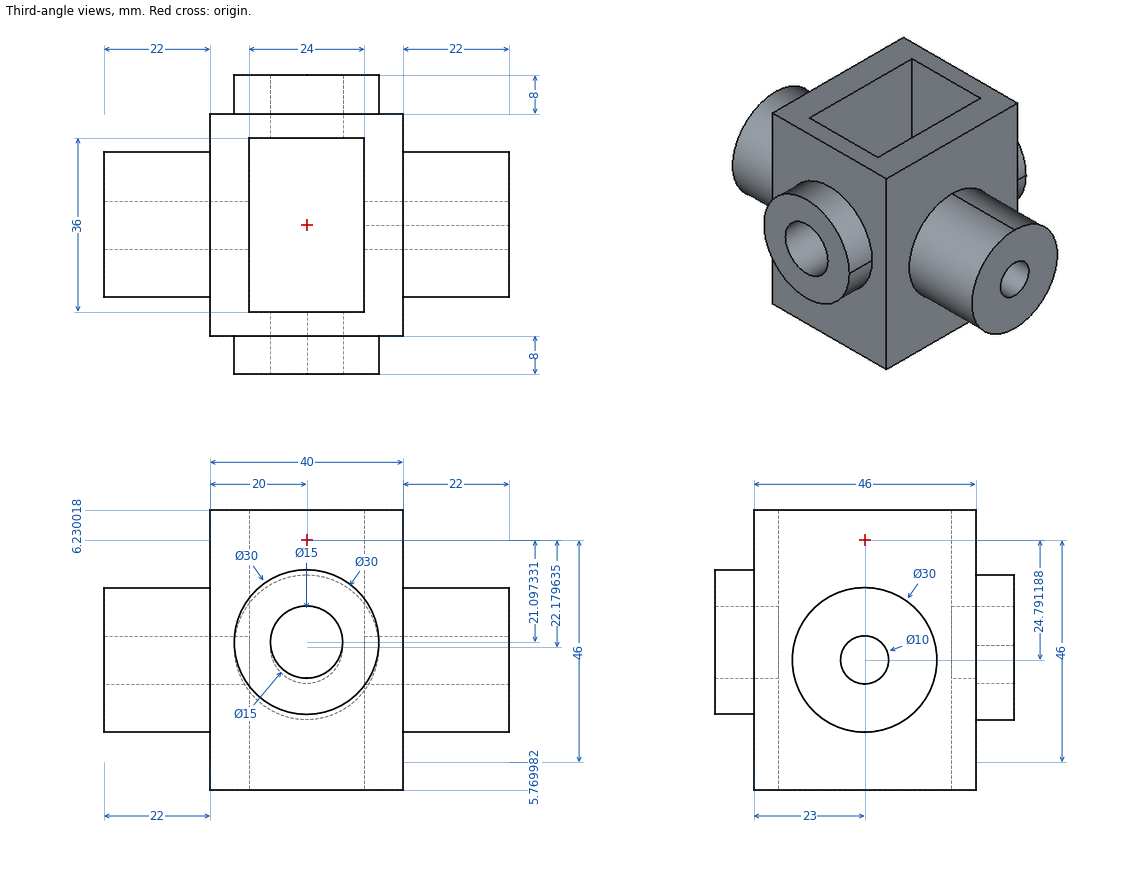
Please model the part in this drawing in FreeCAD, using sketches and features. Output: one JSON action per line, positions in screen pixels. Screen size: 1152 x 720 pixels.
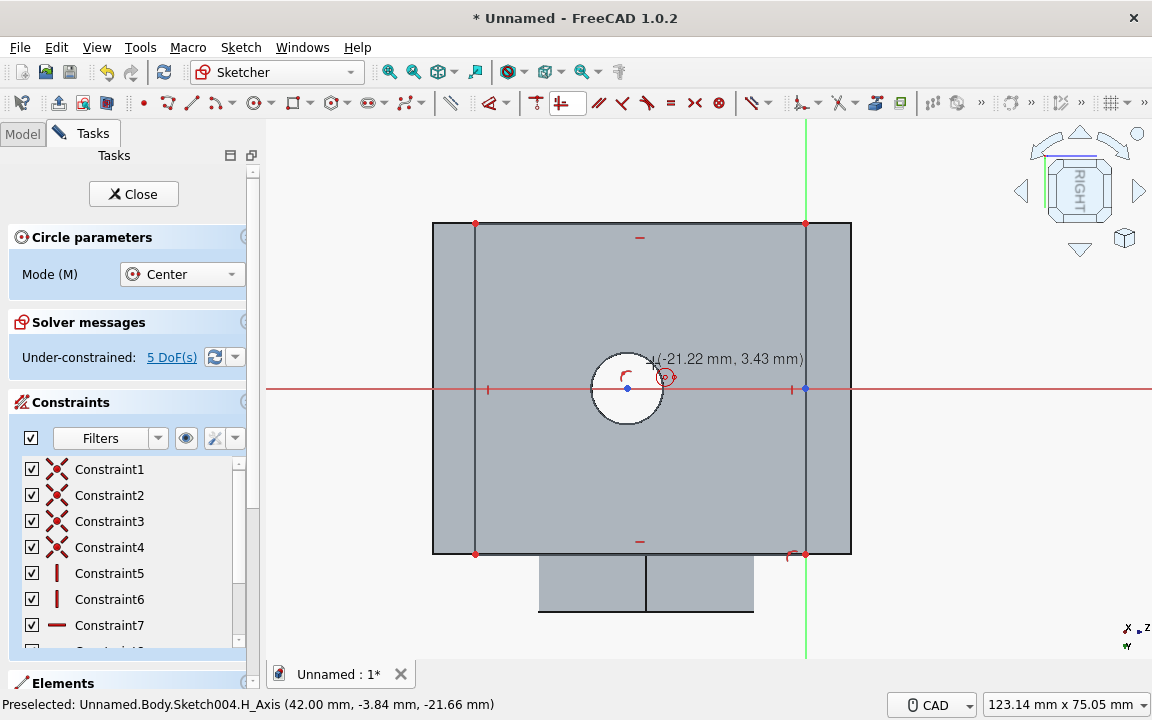
{"action": "left_click", "coordinate": [627, 389]}
{"action": "left_click", "coordinate": [704, 312]}
{"action": "key", "text": "Escape"}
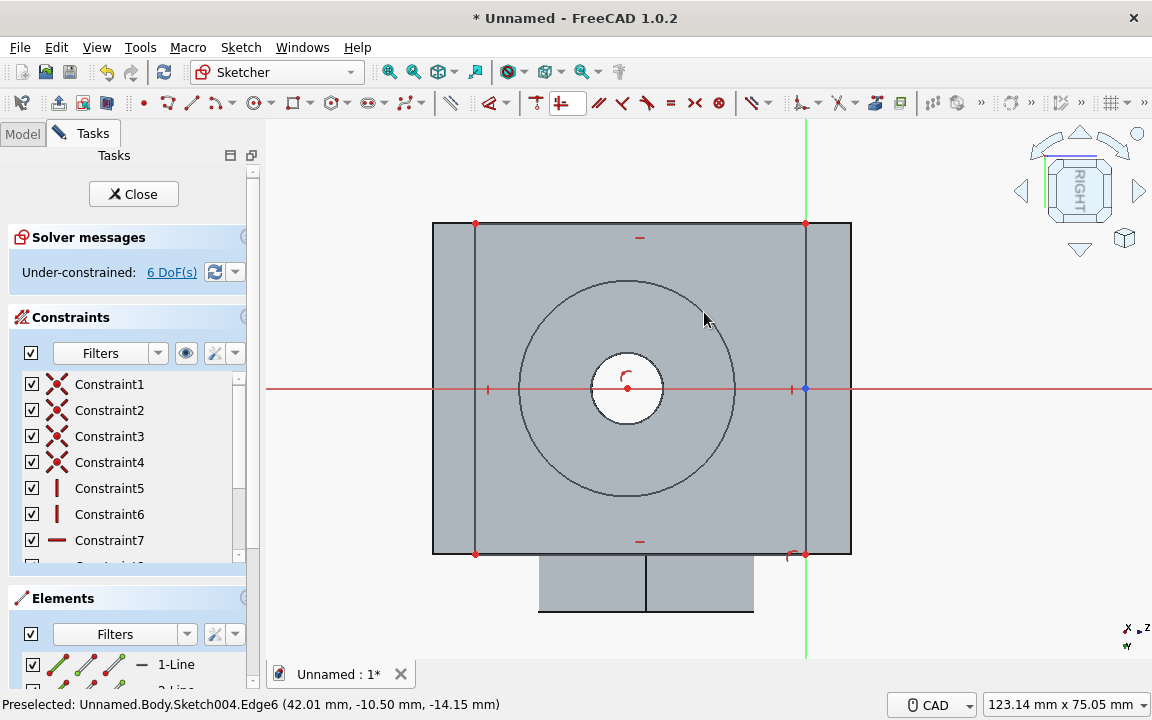
{"action": "left_click", "coordinate": [490, 104]}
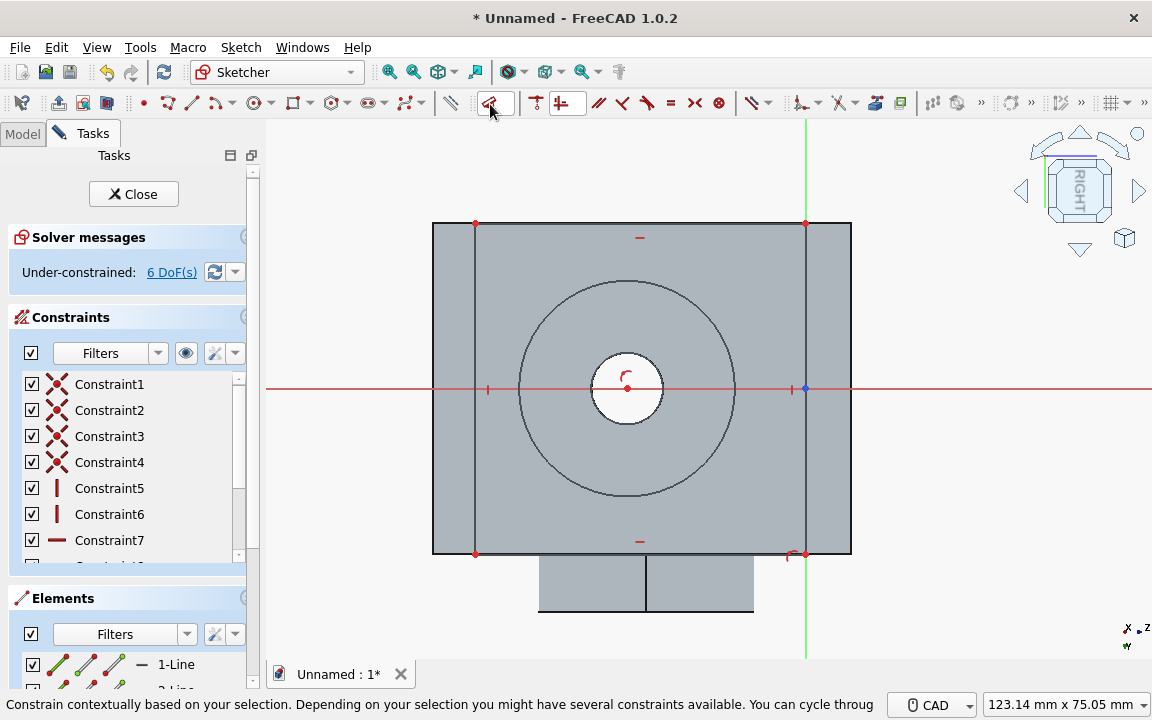
{"action": "left_click", "coordinate": [652, 363]}
{"action": "left_click", "coordinate": [674, 340]}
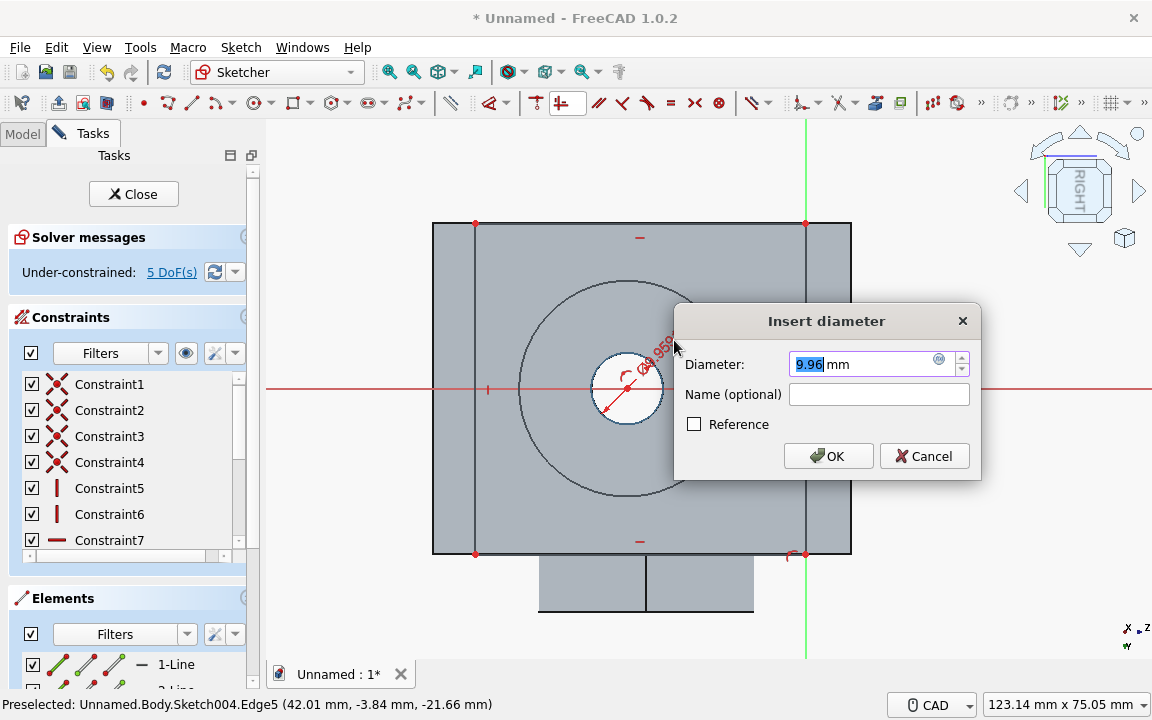
{"action": "type", "text": "10"}
{"action": "key", "text": "Return"}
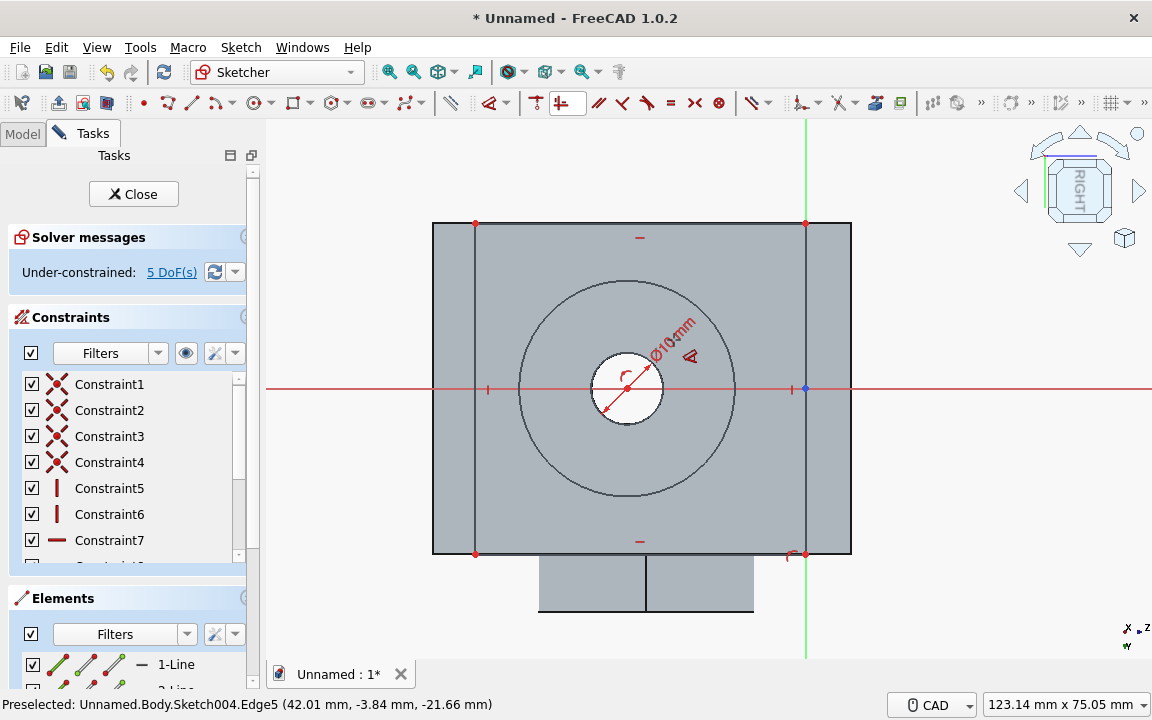
{"action": "left_click", "coordinate": [703, 312]}
{"action": "left_click", "coordinate": [726, 289]}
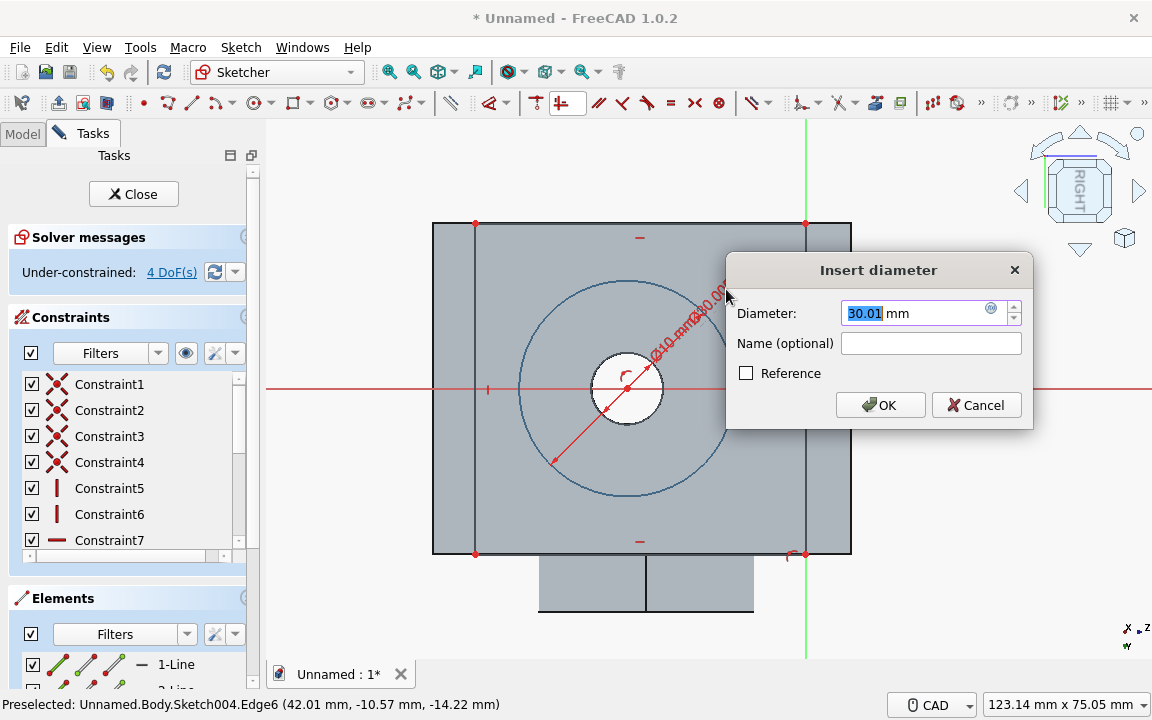
{"action": "type", "text": "30"}
{"action": "key", "text": "Return"}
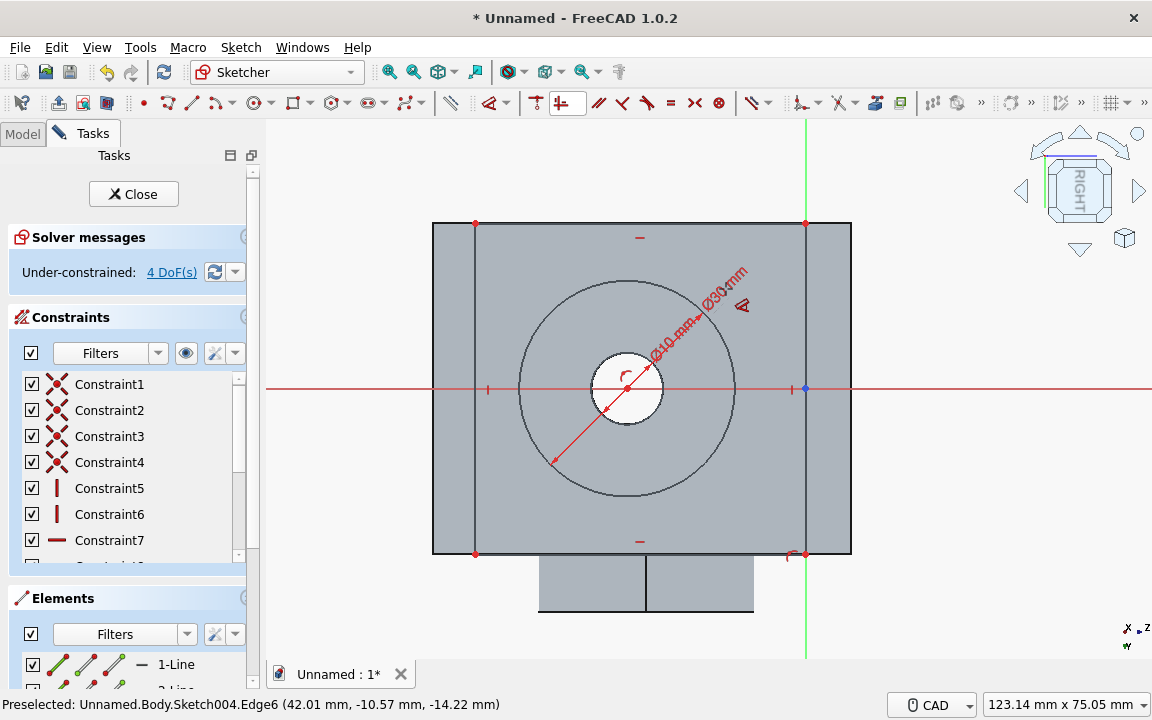
{"action": "left_click", "coordinate": [475, 323]}
{"action": "left_click", "coordinate": [441, 313]}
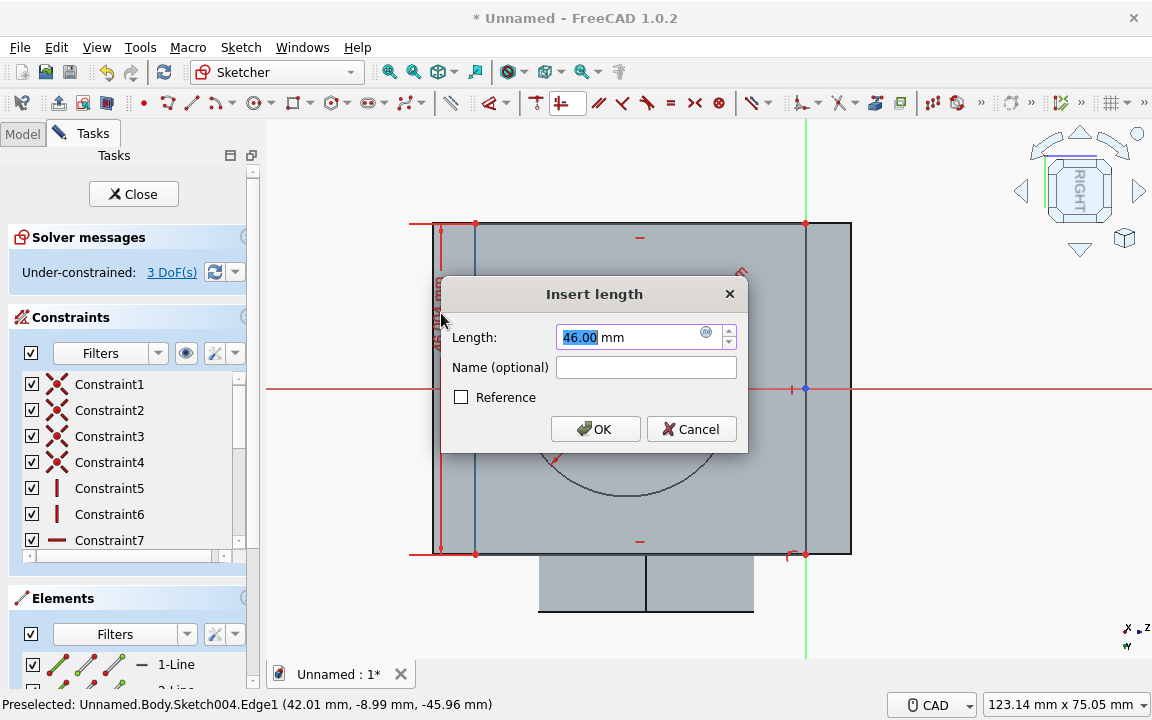
{"action": "type", "text": "46"}
{"action": "key", "text": "Return"}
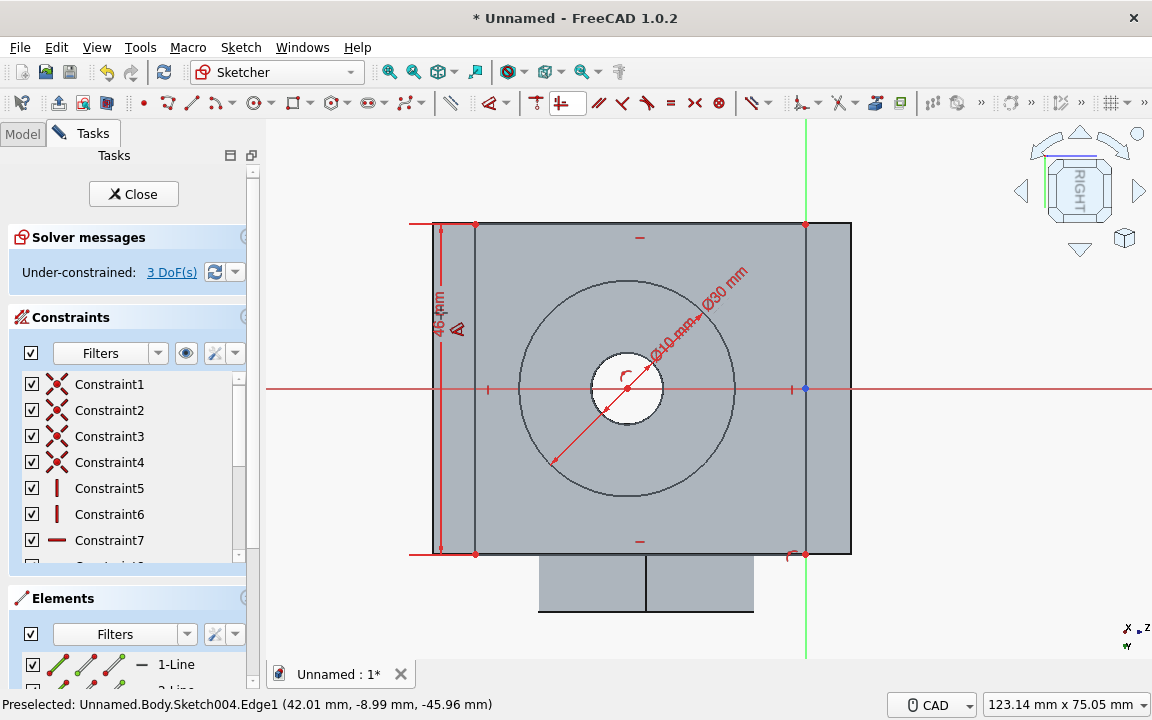
{"action": "left_click", "coordinate": [574, 555]}
{"action": "left_click", "coordinate": [640, 589]}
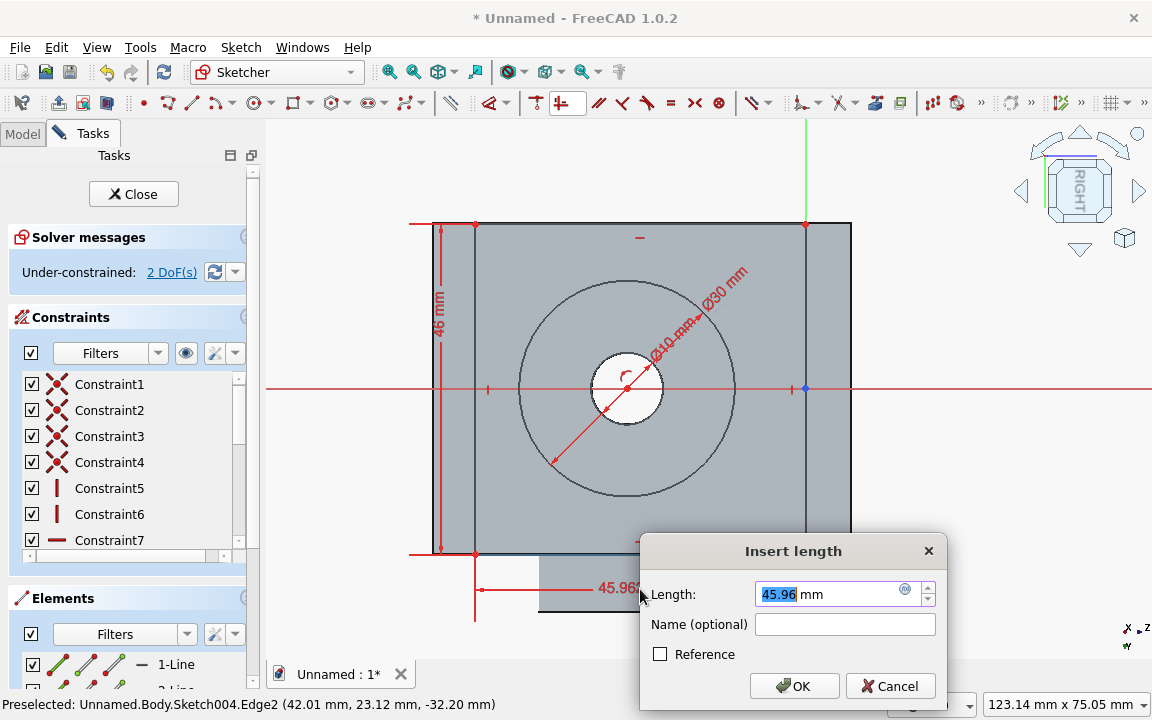
{"action": "type", "text": "46"}
{"action": "key", "text": "Return"}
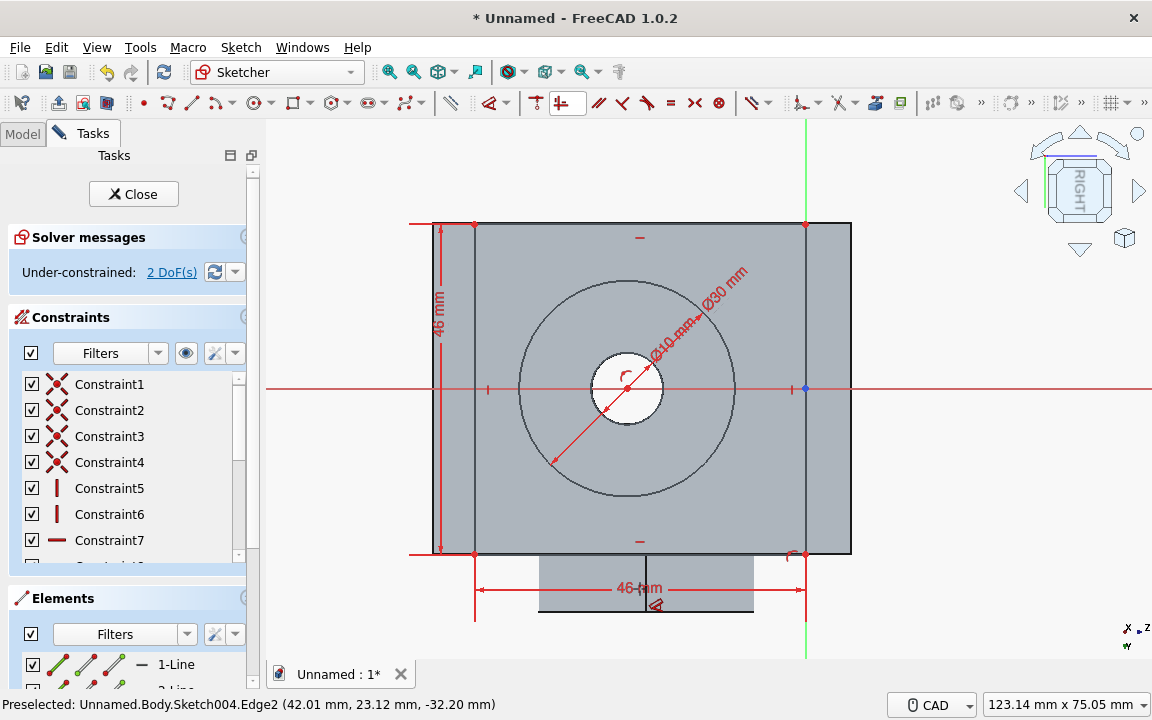
{"action": "left_click", "coordinate": [475, 224]}
{"action": "left_click", "coordinate": [840, 306]}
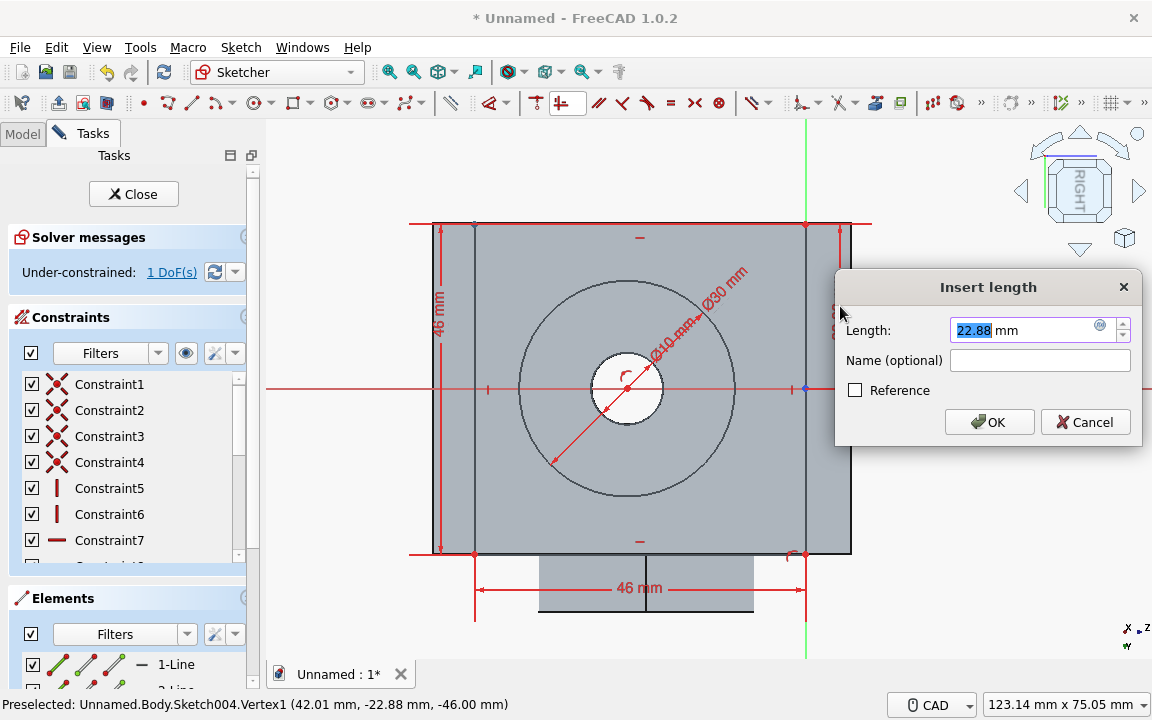
{"action": "type", "text": "23"}
{"action": "key", "text": "Return"}